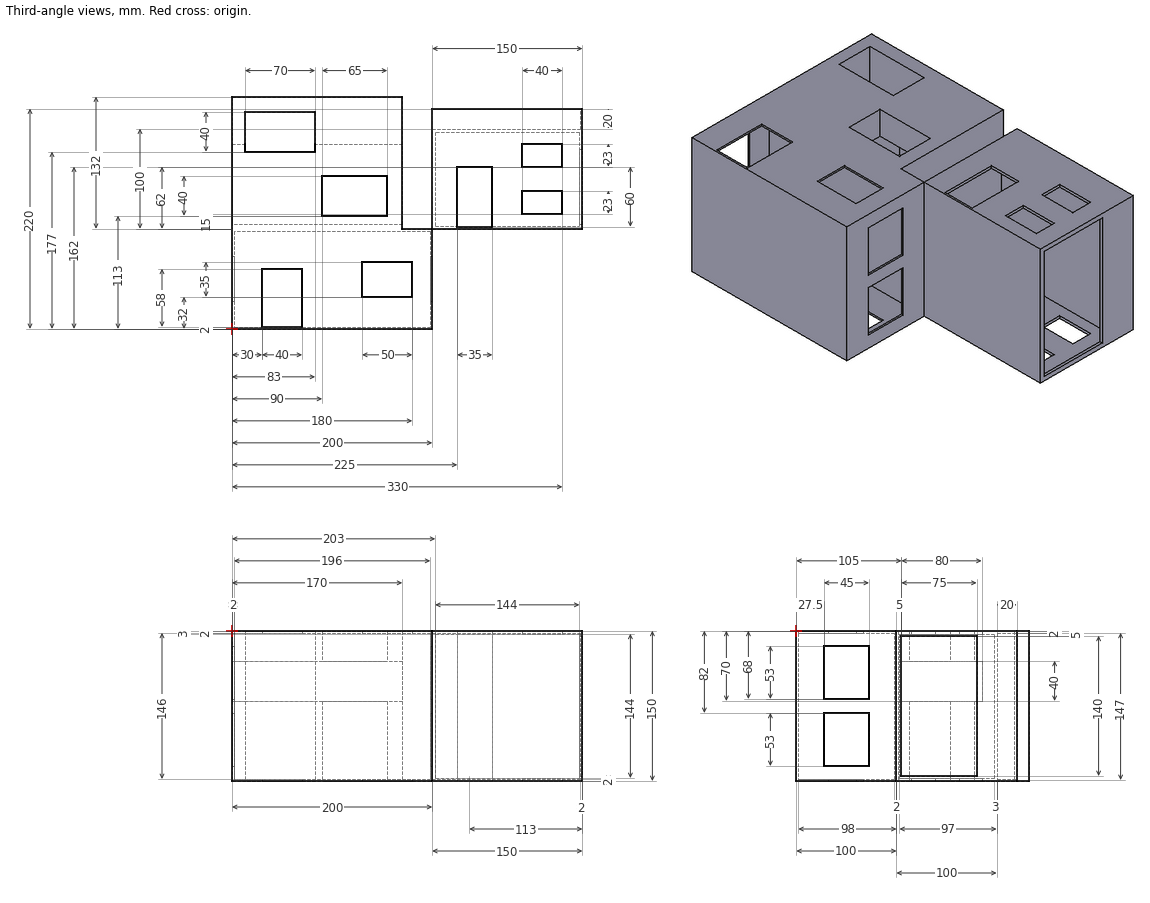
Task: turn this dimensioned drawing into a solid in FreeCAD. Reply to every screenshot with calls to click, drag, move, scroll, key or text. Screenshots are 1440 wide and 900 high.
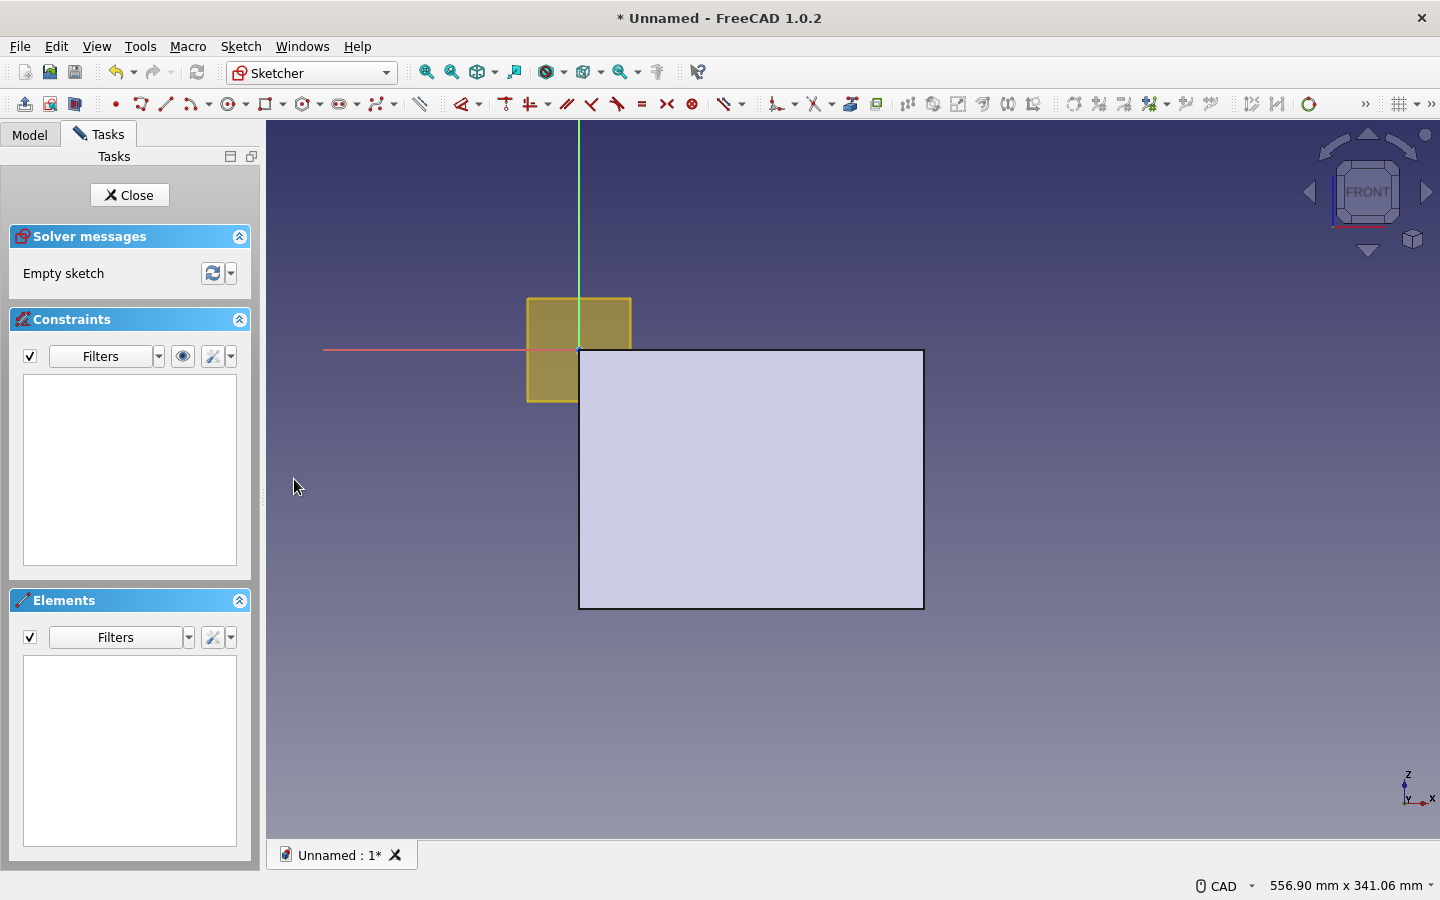
click(264, 104)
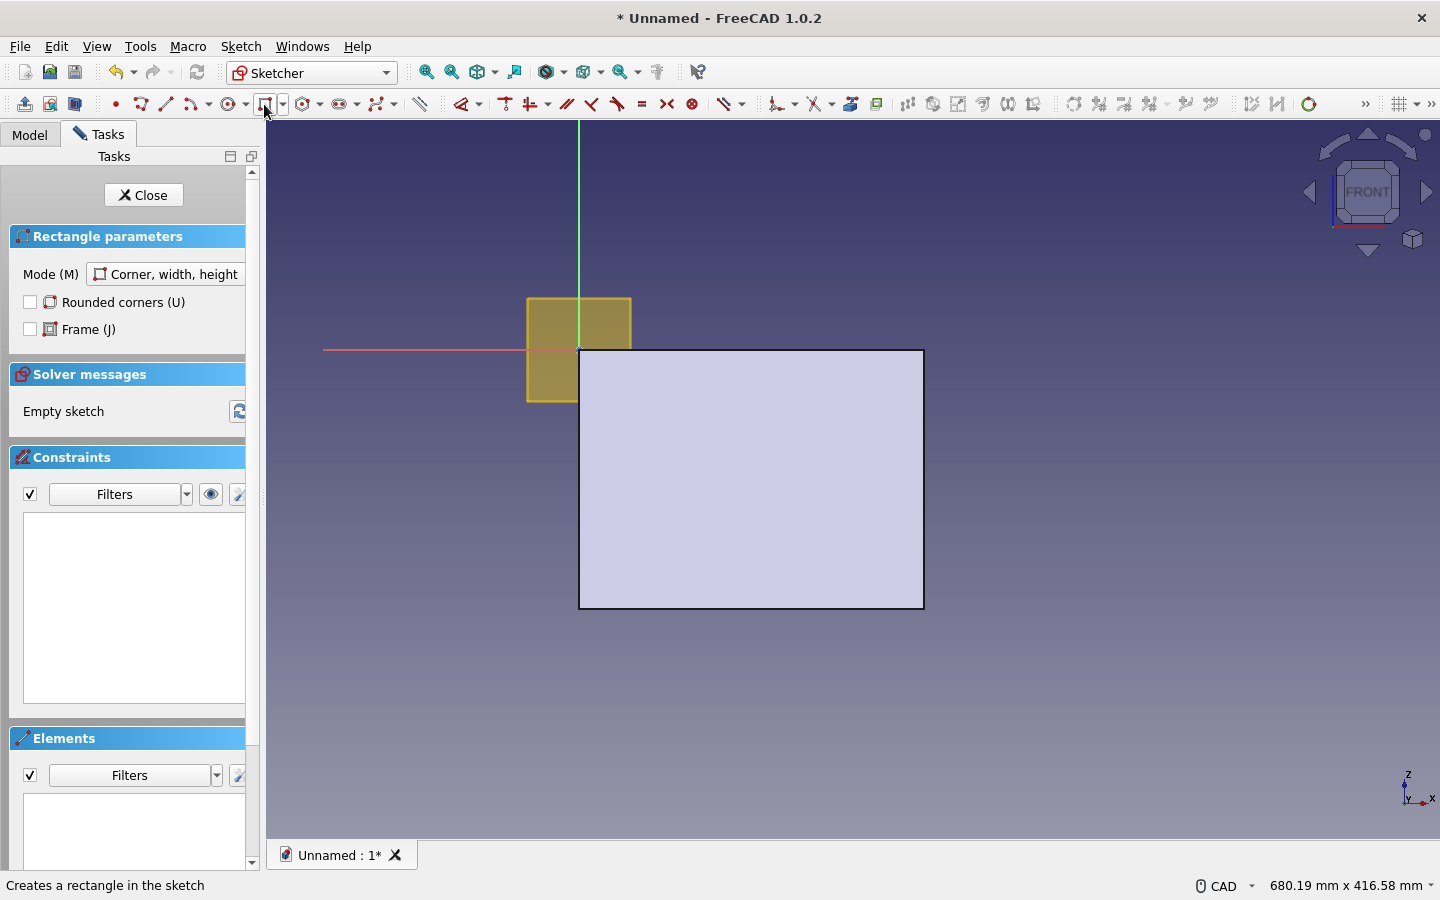
click(924, 350)
move(1183, 609)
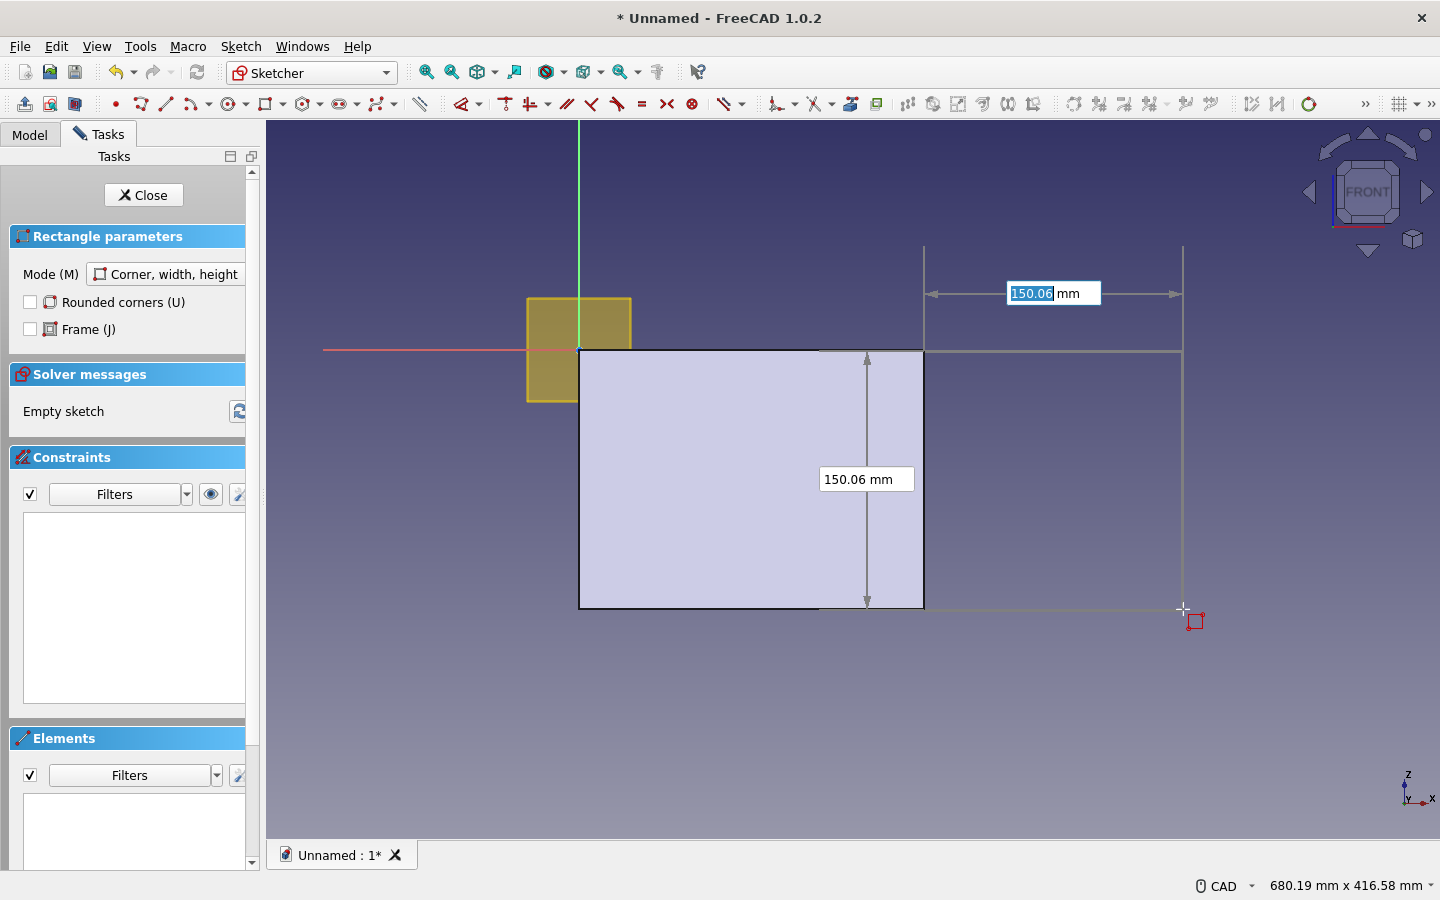
text(150)
key(Tab)
text(150)
key(Return)
key(Escape)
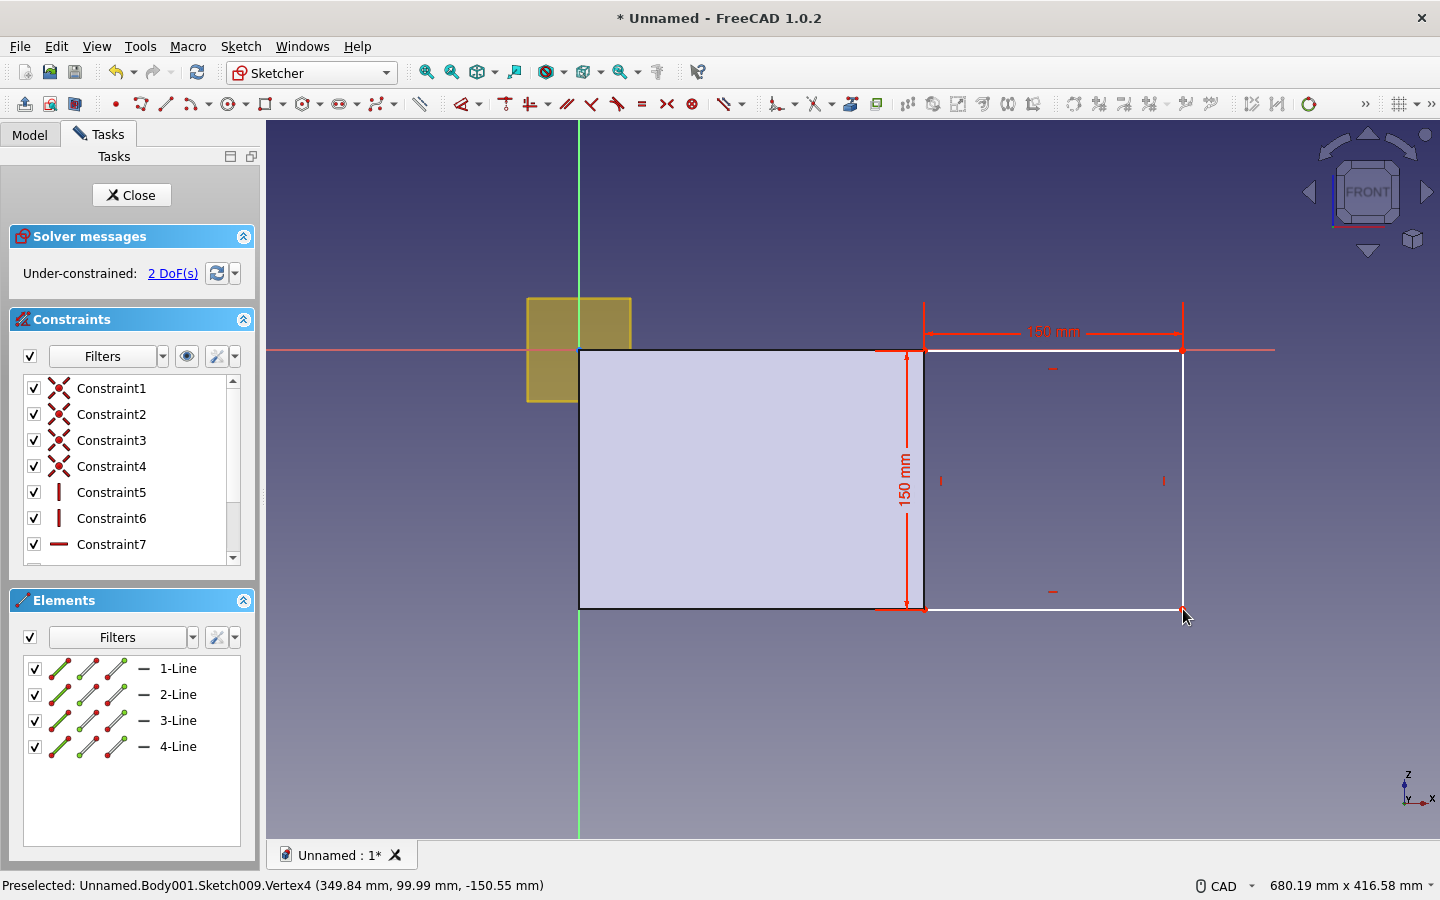
click(924, 351)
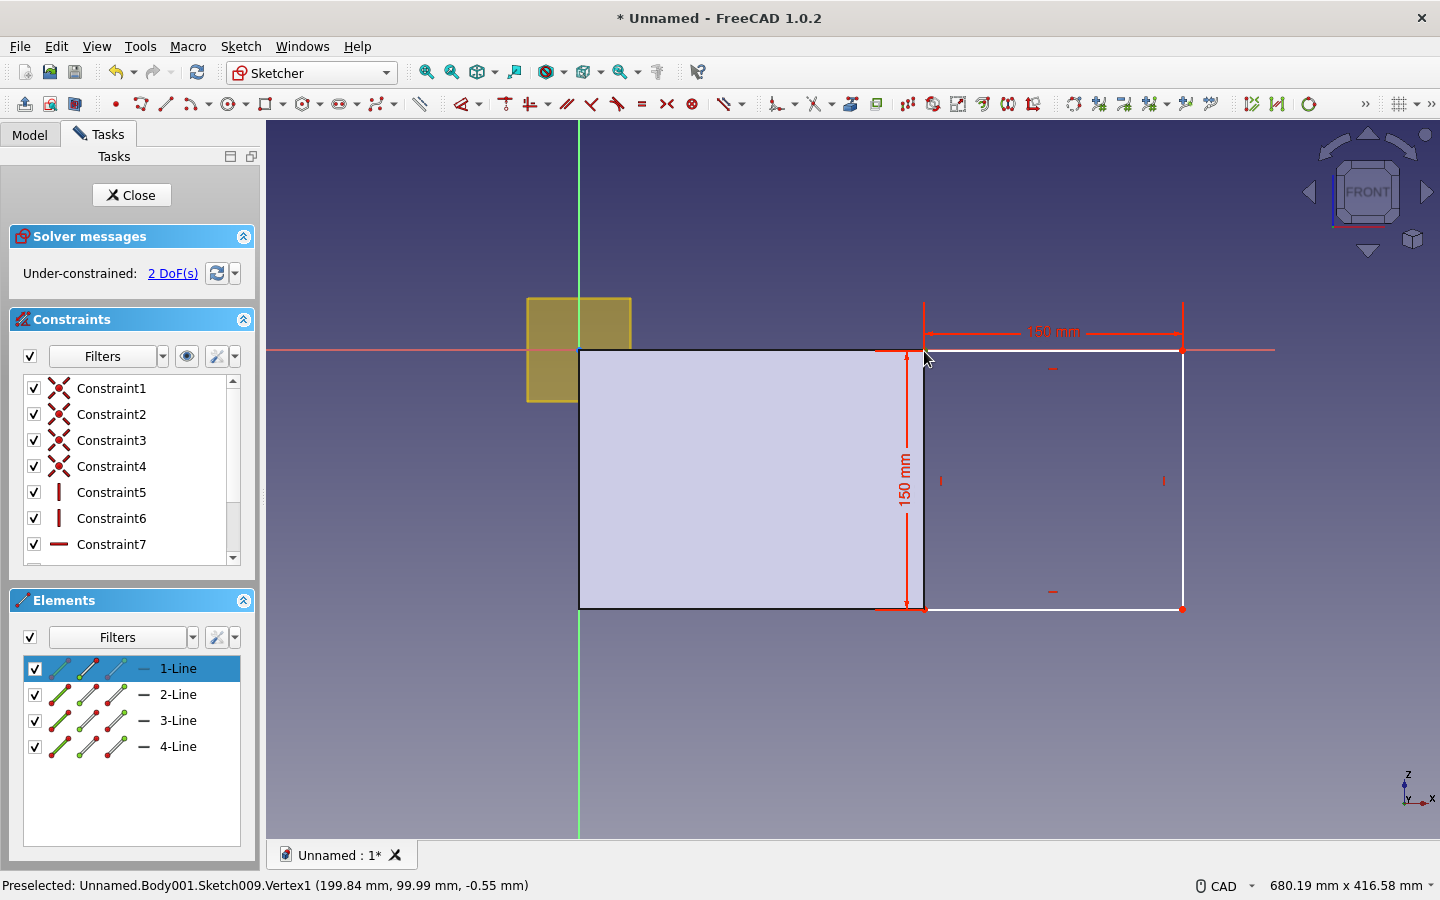
click(364, 350)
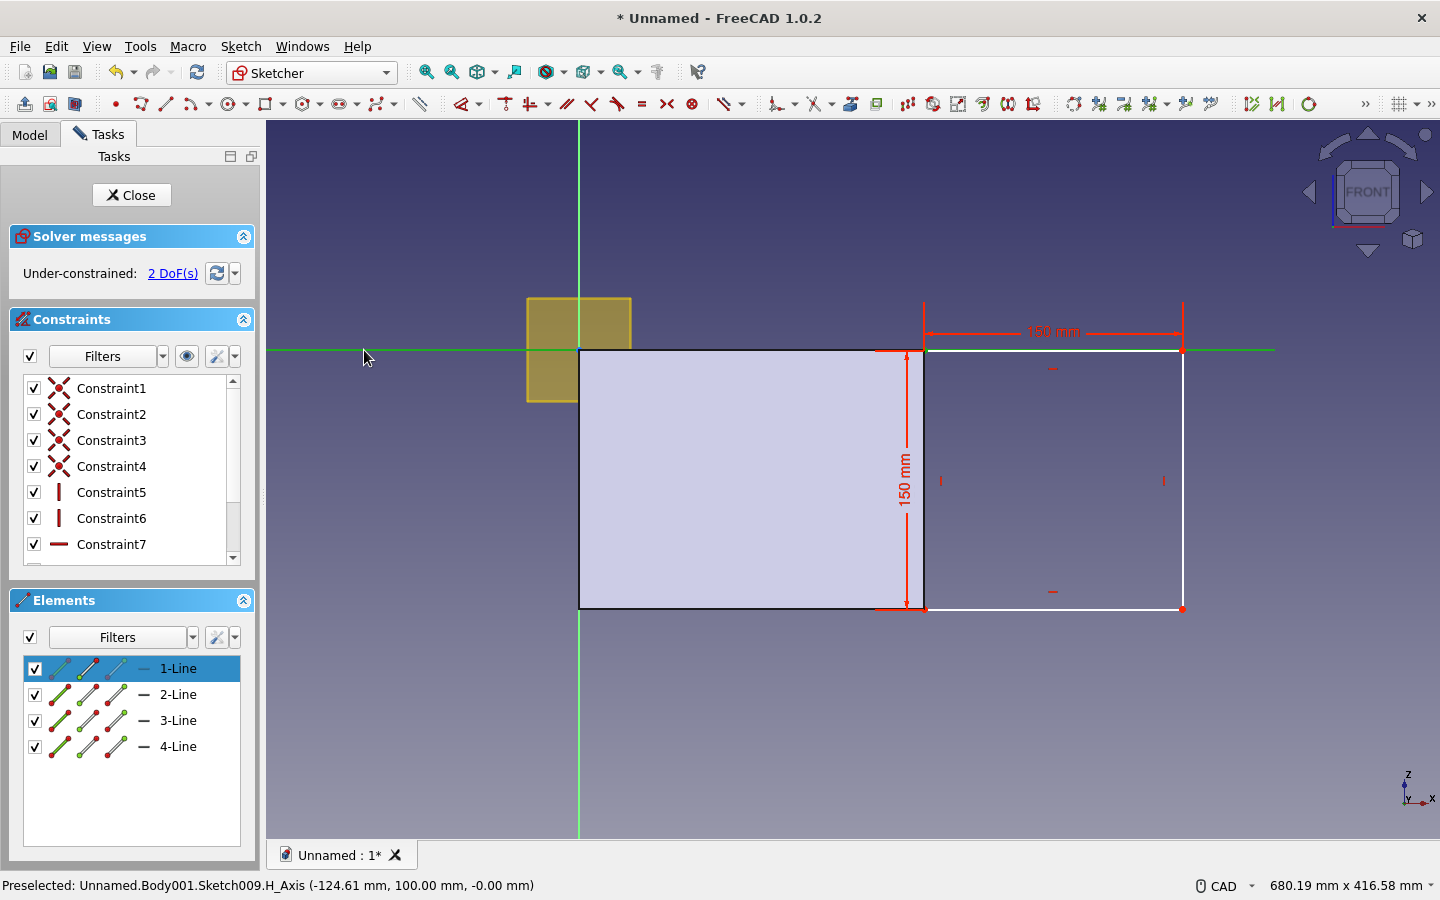
click(505, 104)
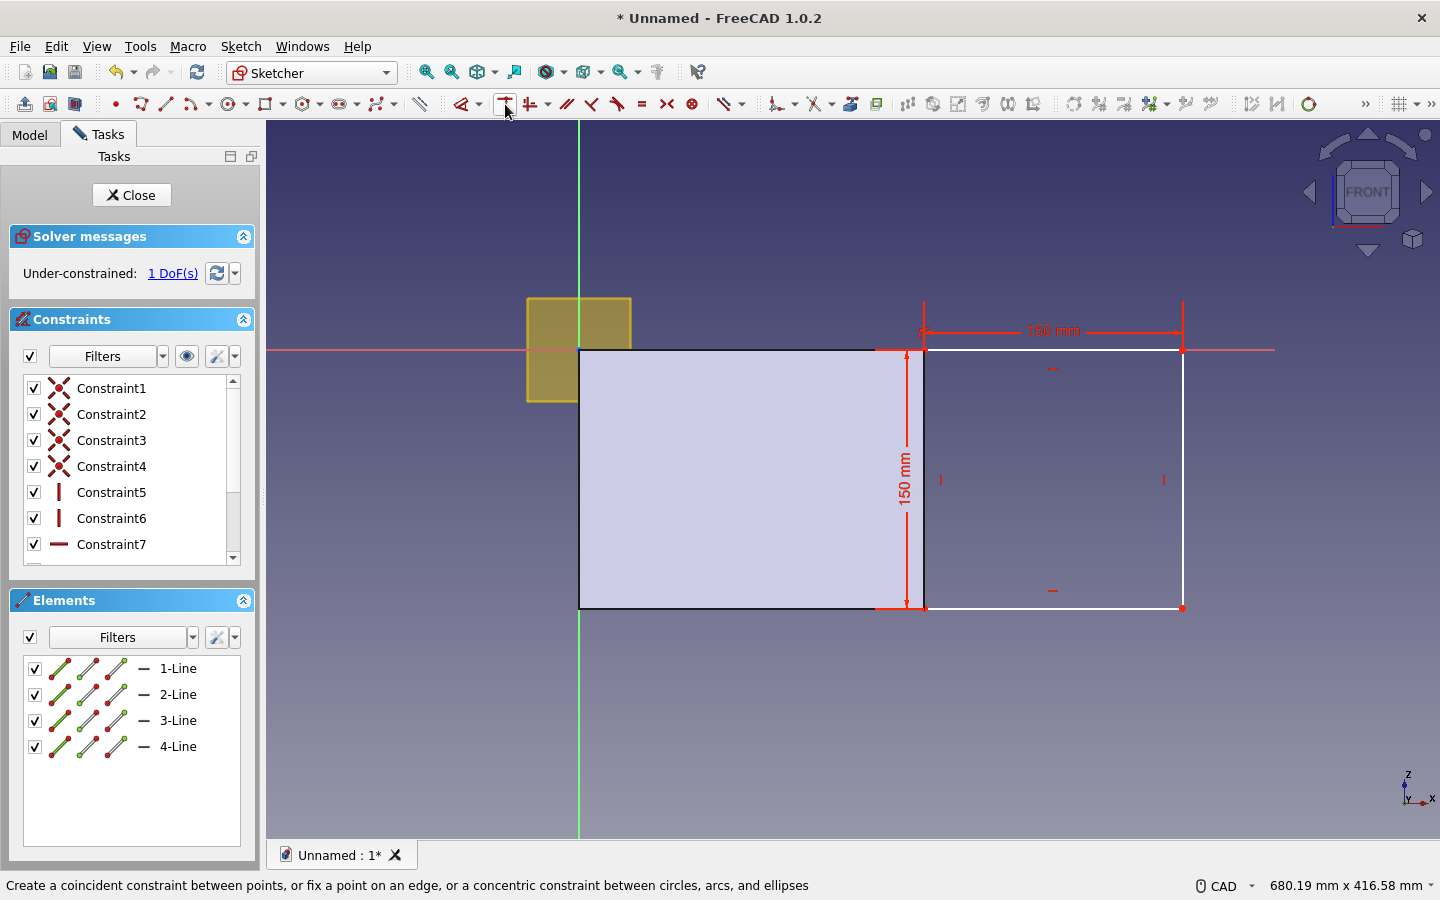
click(460, 104)